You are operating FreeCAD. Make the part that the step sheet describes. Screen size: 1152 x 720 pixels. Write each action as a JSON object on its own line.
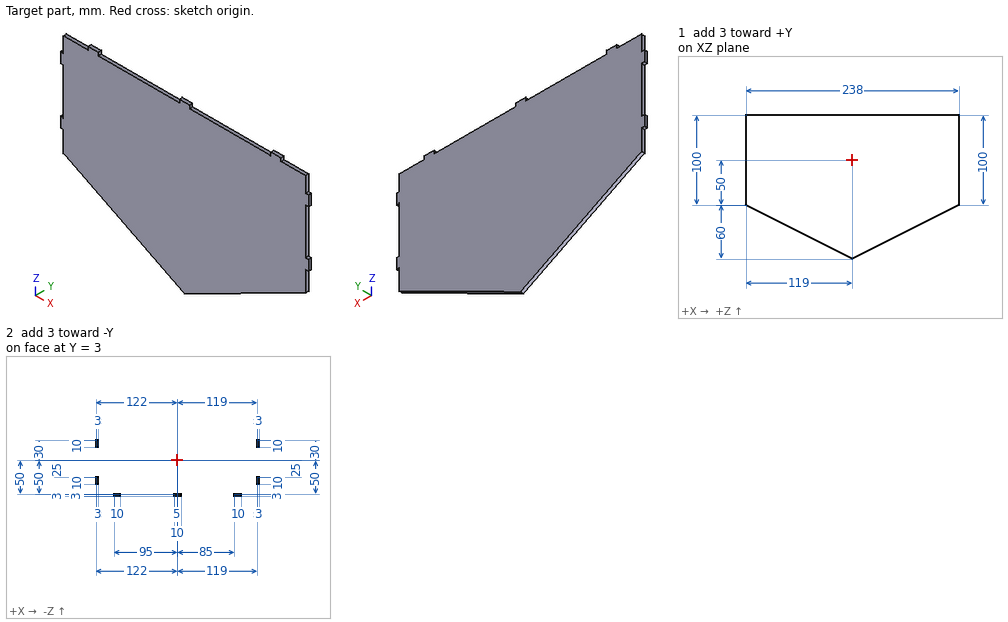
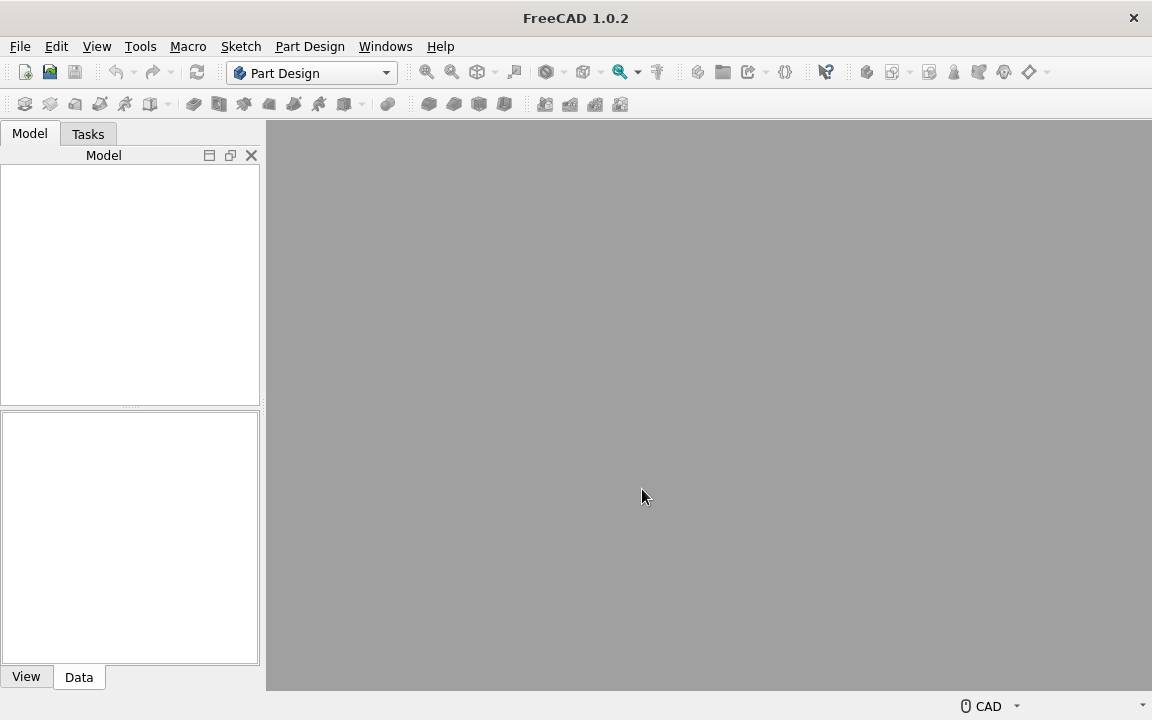
{"action": "left_click", "coordinate": [25, 72]}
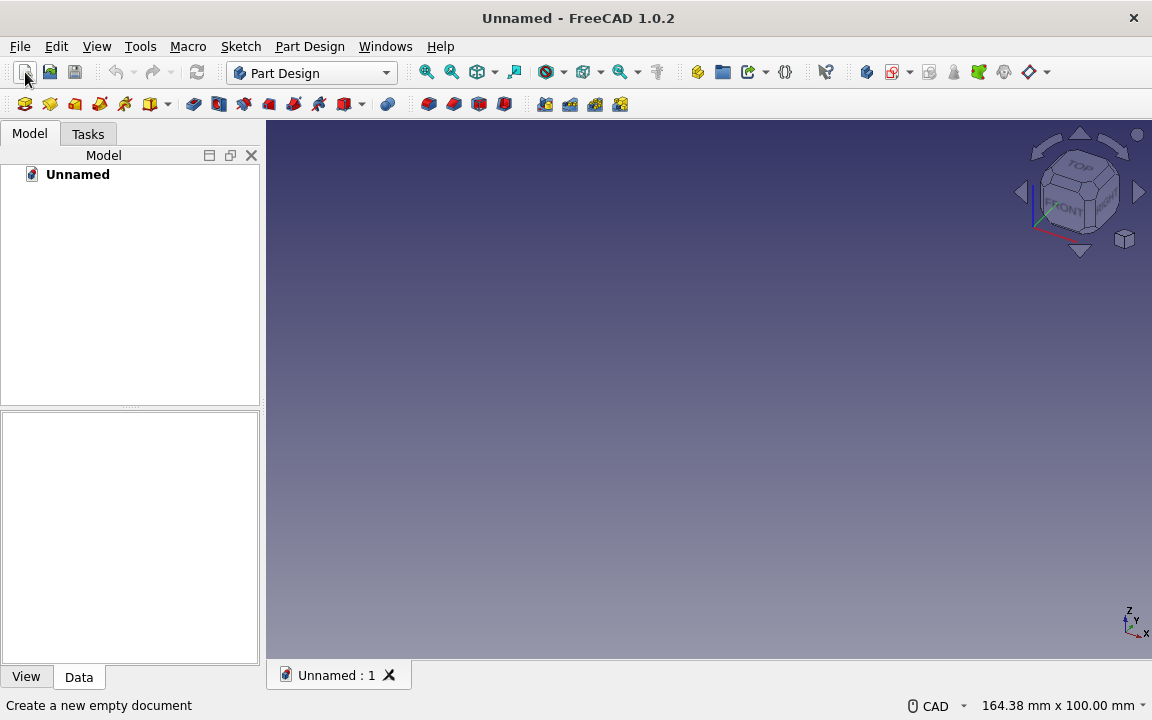
{"action": "left_click", "coordinate": [892, 72]}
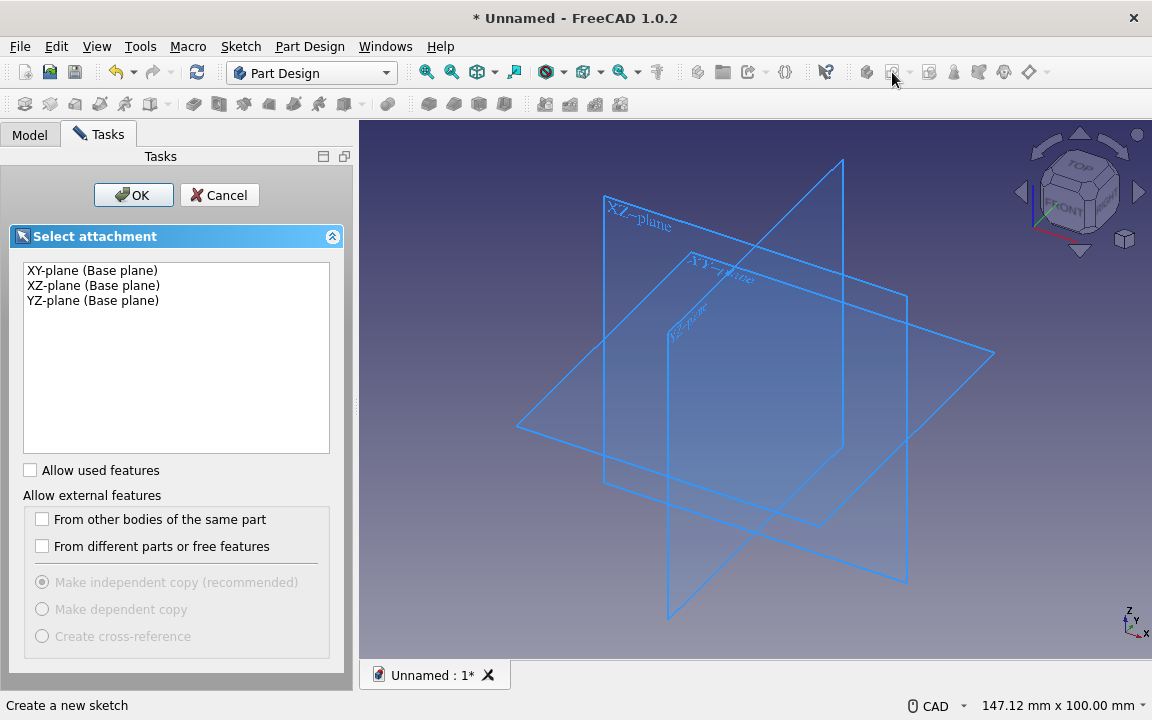
{"action": "left_click", "coordinate": [84, 286]}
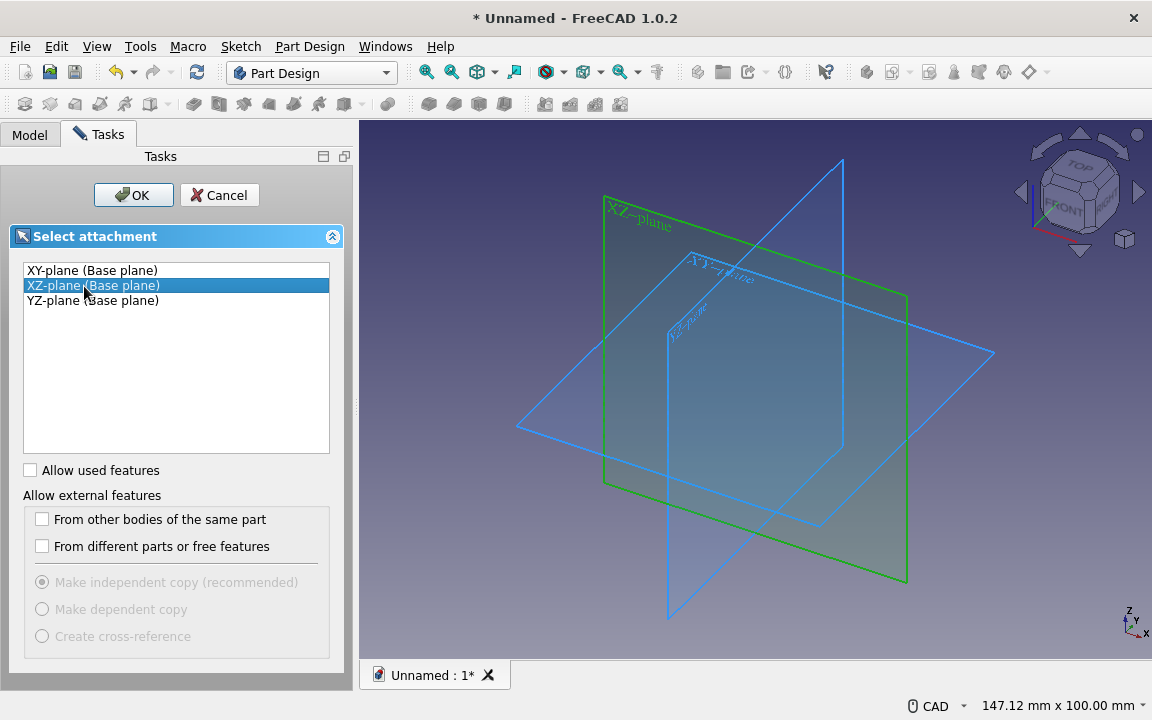
{"action": "left_click", "coordinate": [134, 195]}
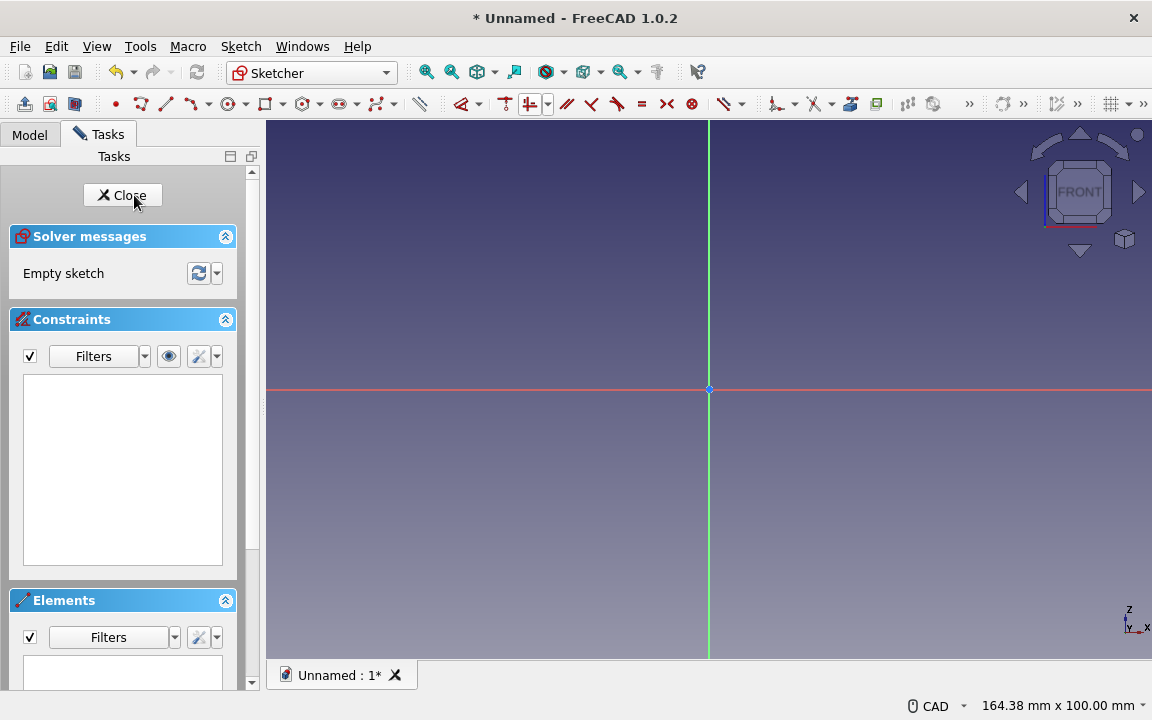
{"action": "scroll", "coordinate": [601, 295], "scroll_direction": "down", "scroll_amount": 5}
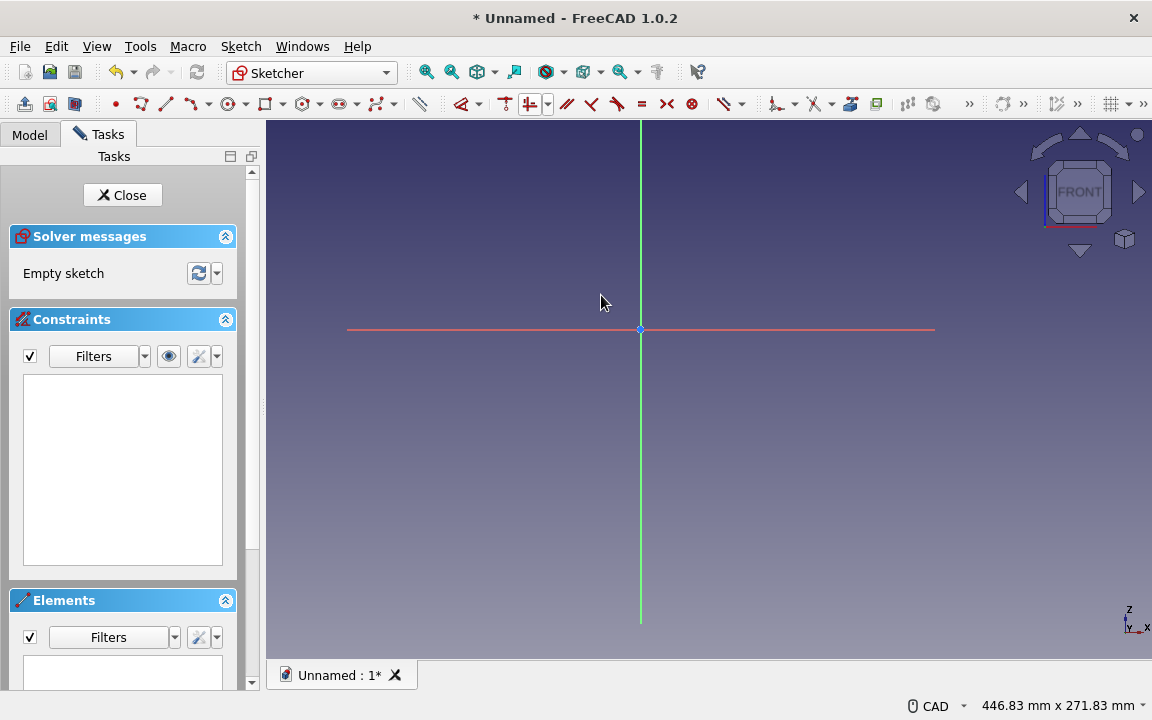
{"action": "key", "text": "g m"}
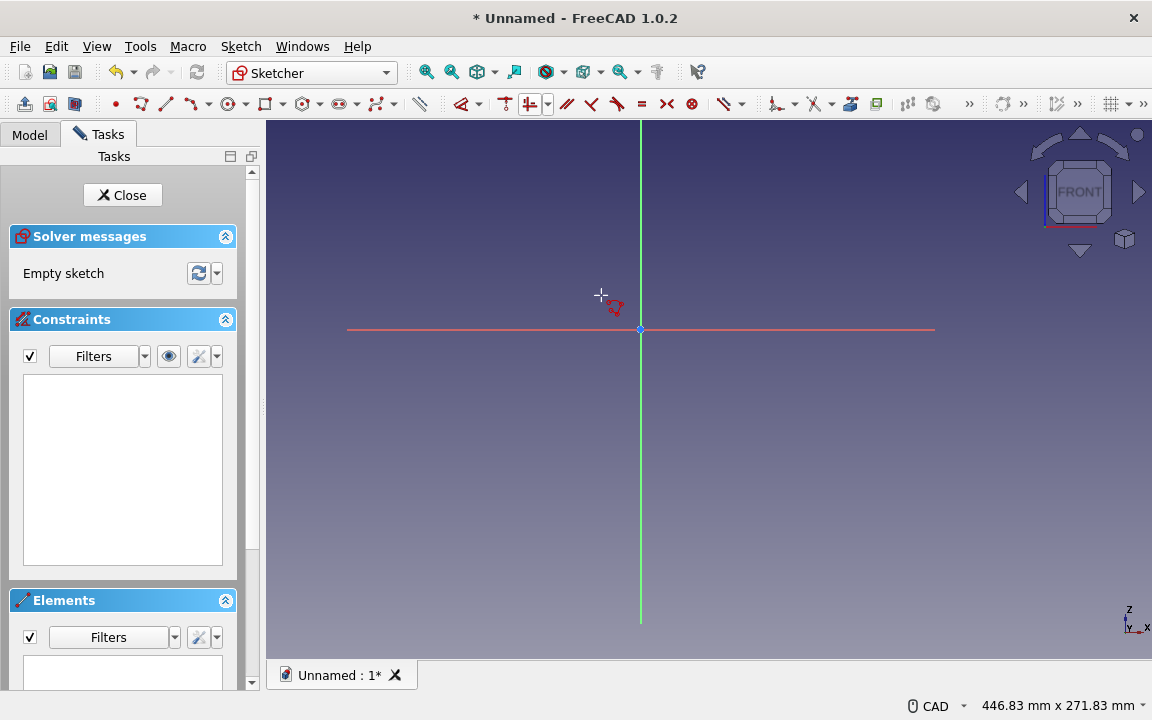
{"action": "left_click", "coordinate": [641, 548]}
{"action": "left_click", "coordinate": [405, 429]}
{"action": "left_click", "coordinate": [405, 231]}
{"action": "left_click", "coordinate": [877, 231]}
{"action": "left_click", "coordinate": [877, 429]}
{"action": "left_click", "coordinate": [641, 549]}
{"action": "key", "text": "Escape"}
{"action": "key", "text": "Escape"}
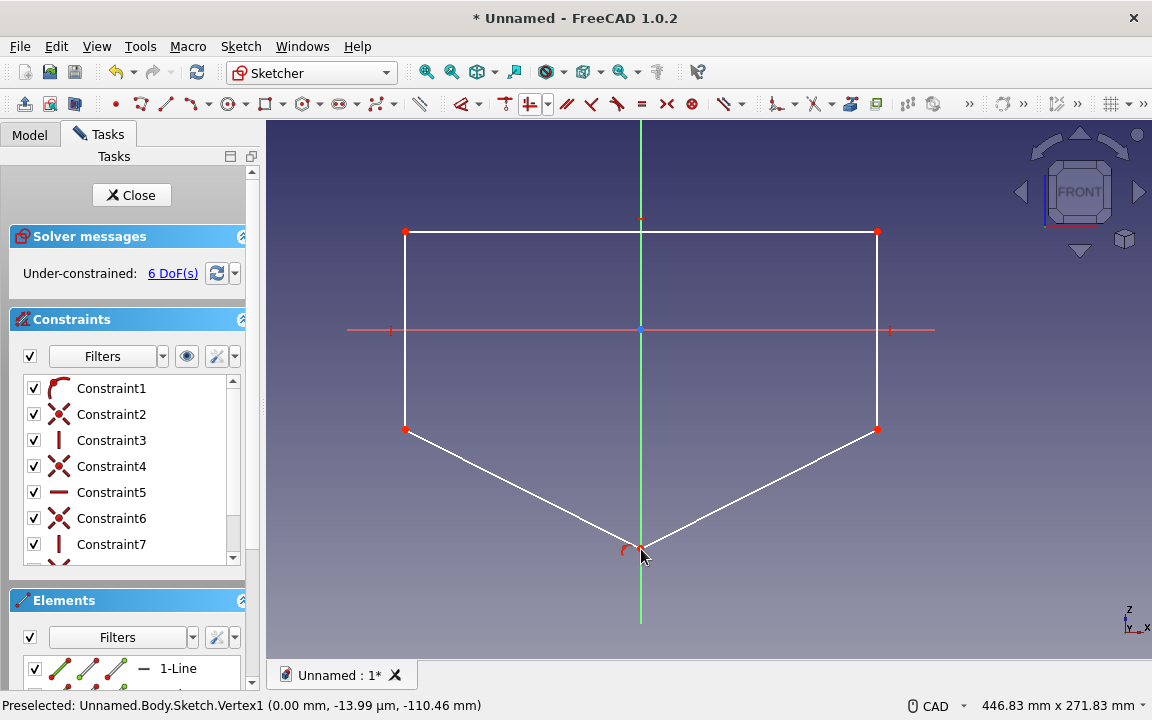
{"action": "left_click", "coordinate": [405, 371]}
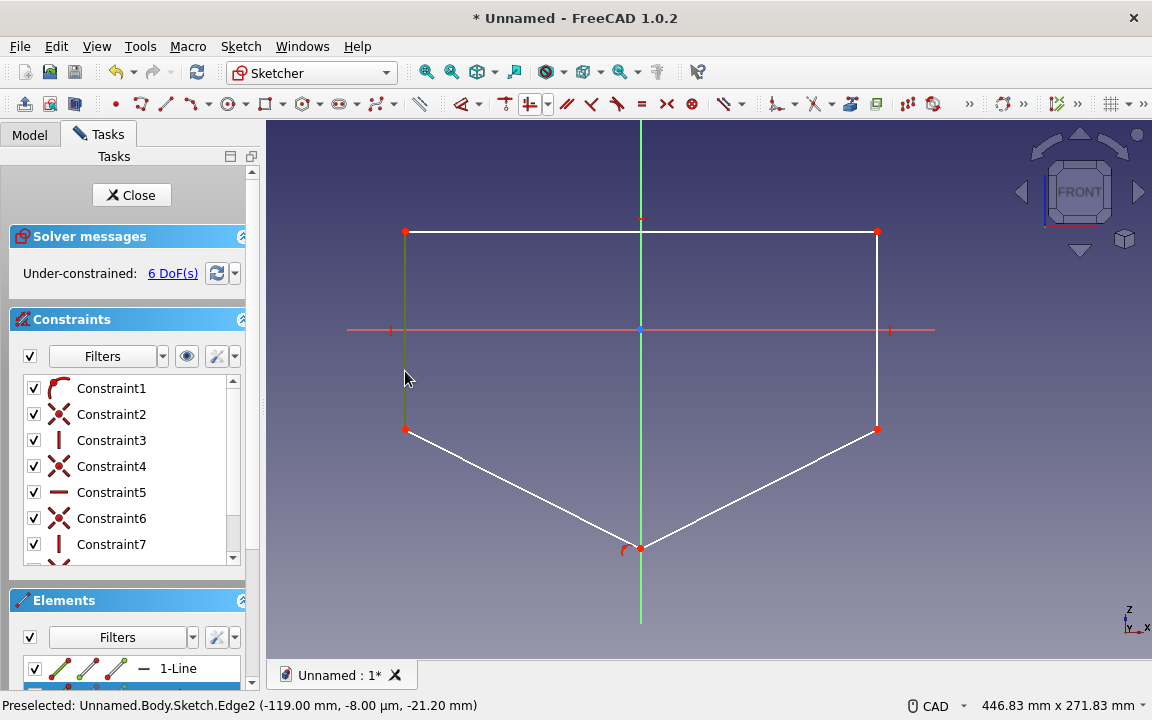
{"action": "key", "text": "i"}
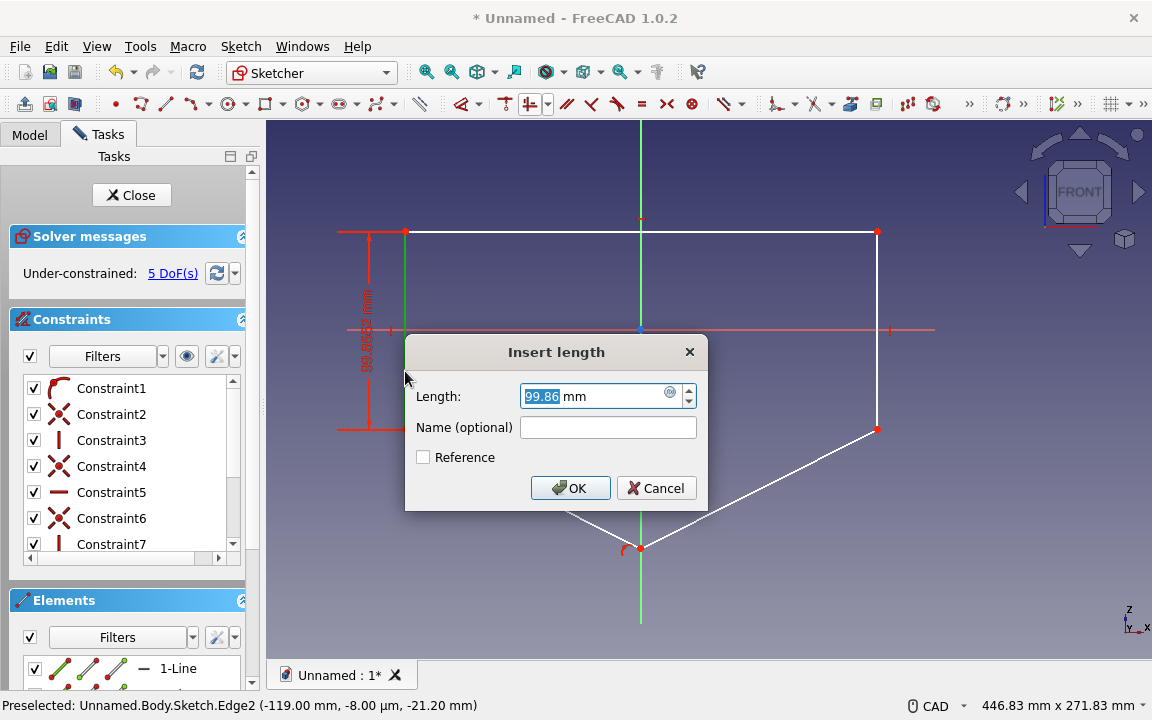
{"action": "type", "text": "100"}
{"action": "key", "text": "Return"}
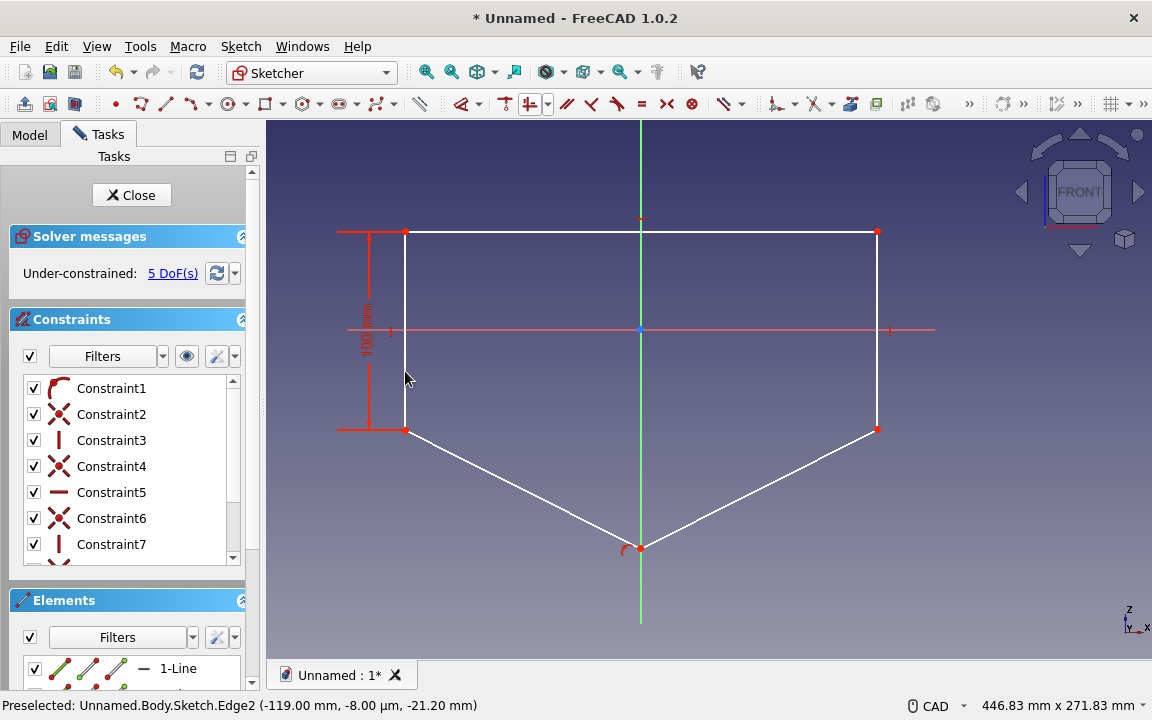
{"action": "left_click", "coordinate": [547, 232]}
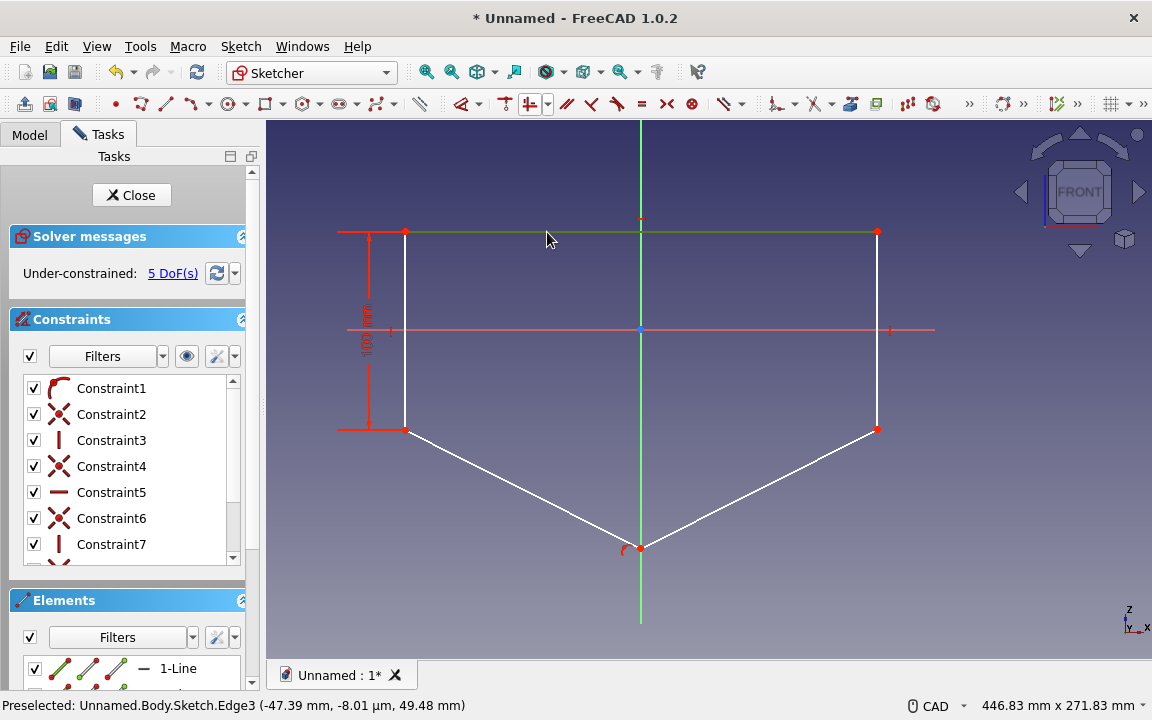
{"action": "key", "text": "l"}